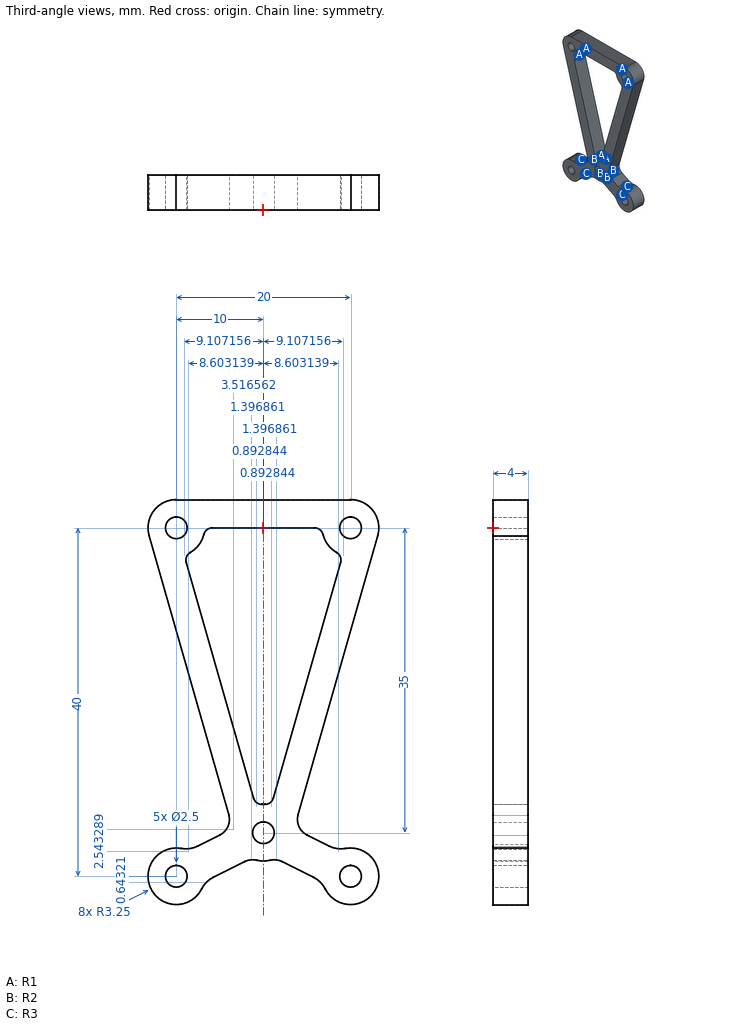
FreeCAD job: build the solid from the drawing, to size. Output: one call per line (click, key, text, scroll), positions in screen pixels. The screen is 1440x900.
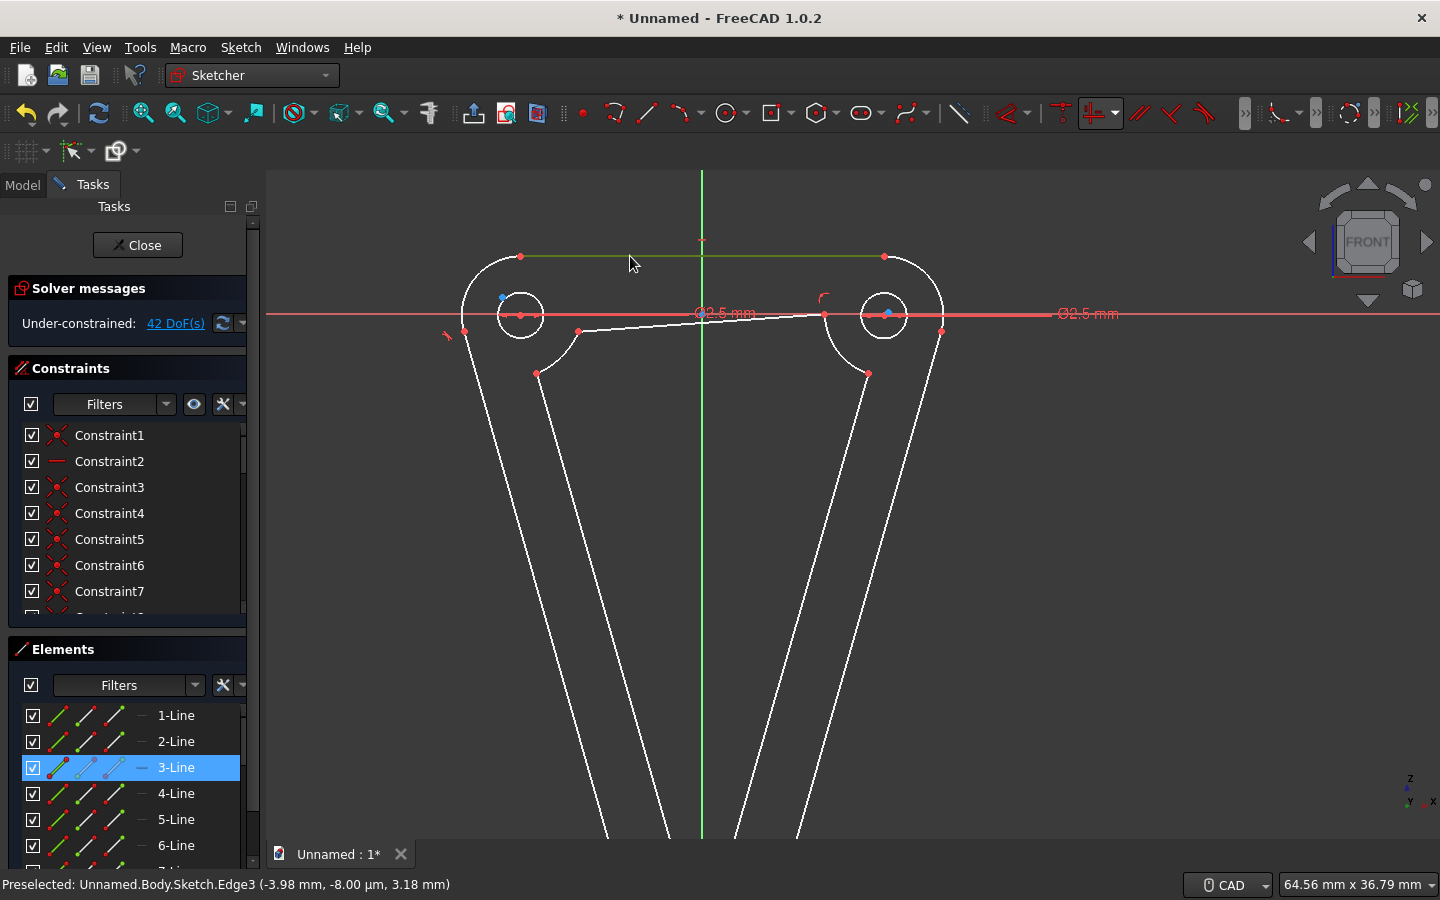
click(490, 265)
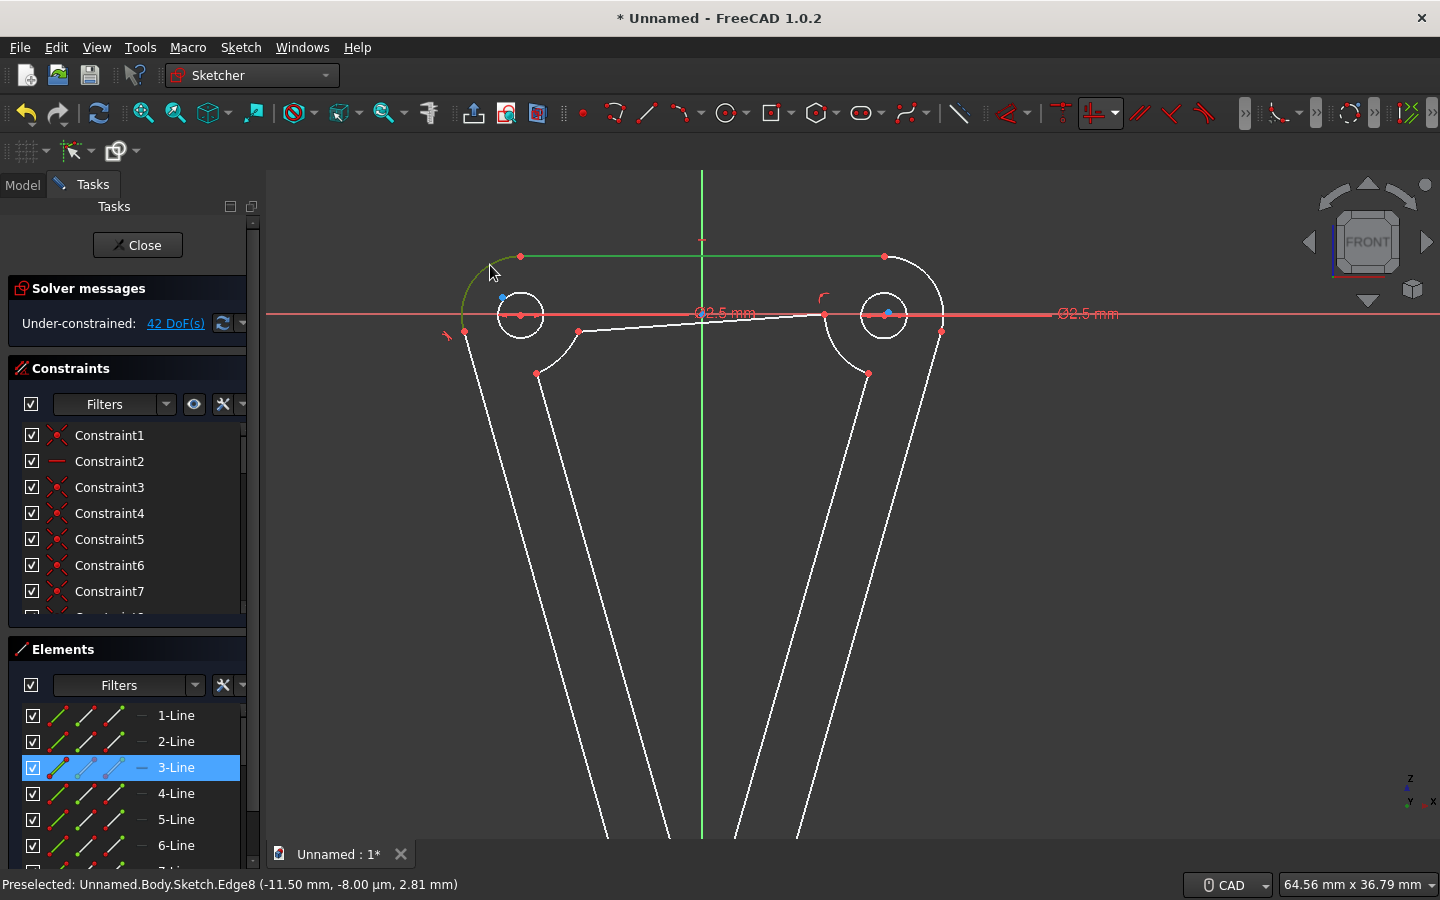
click(1204, 114)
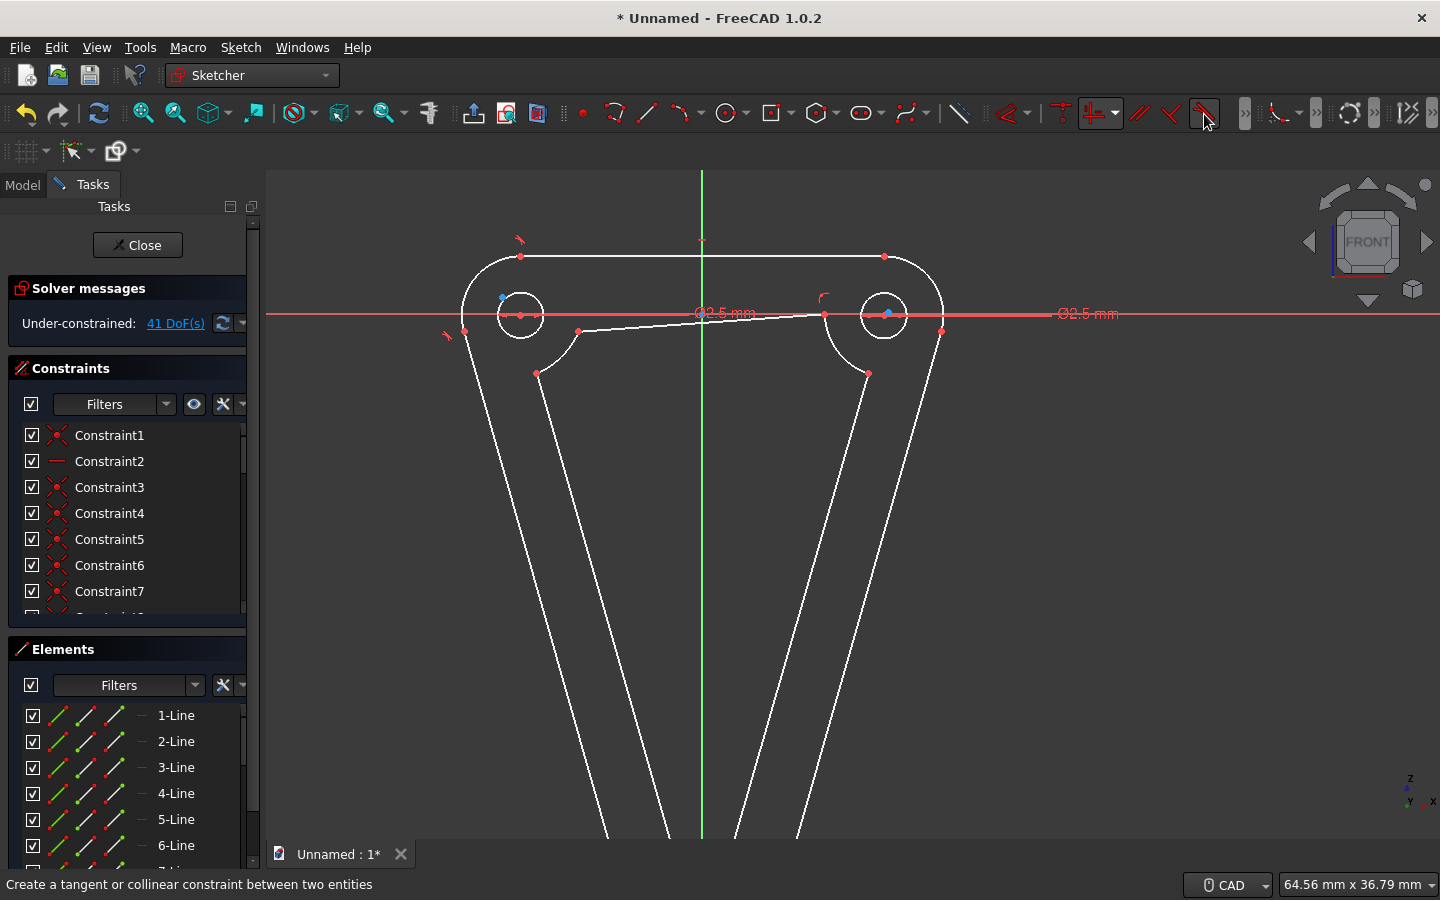
click(630, 256)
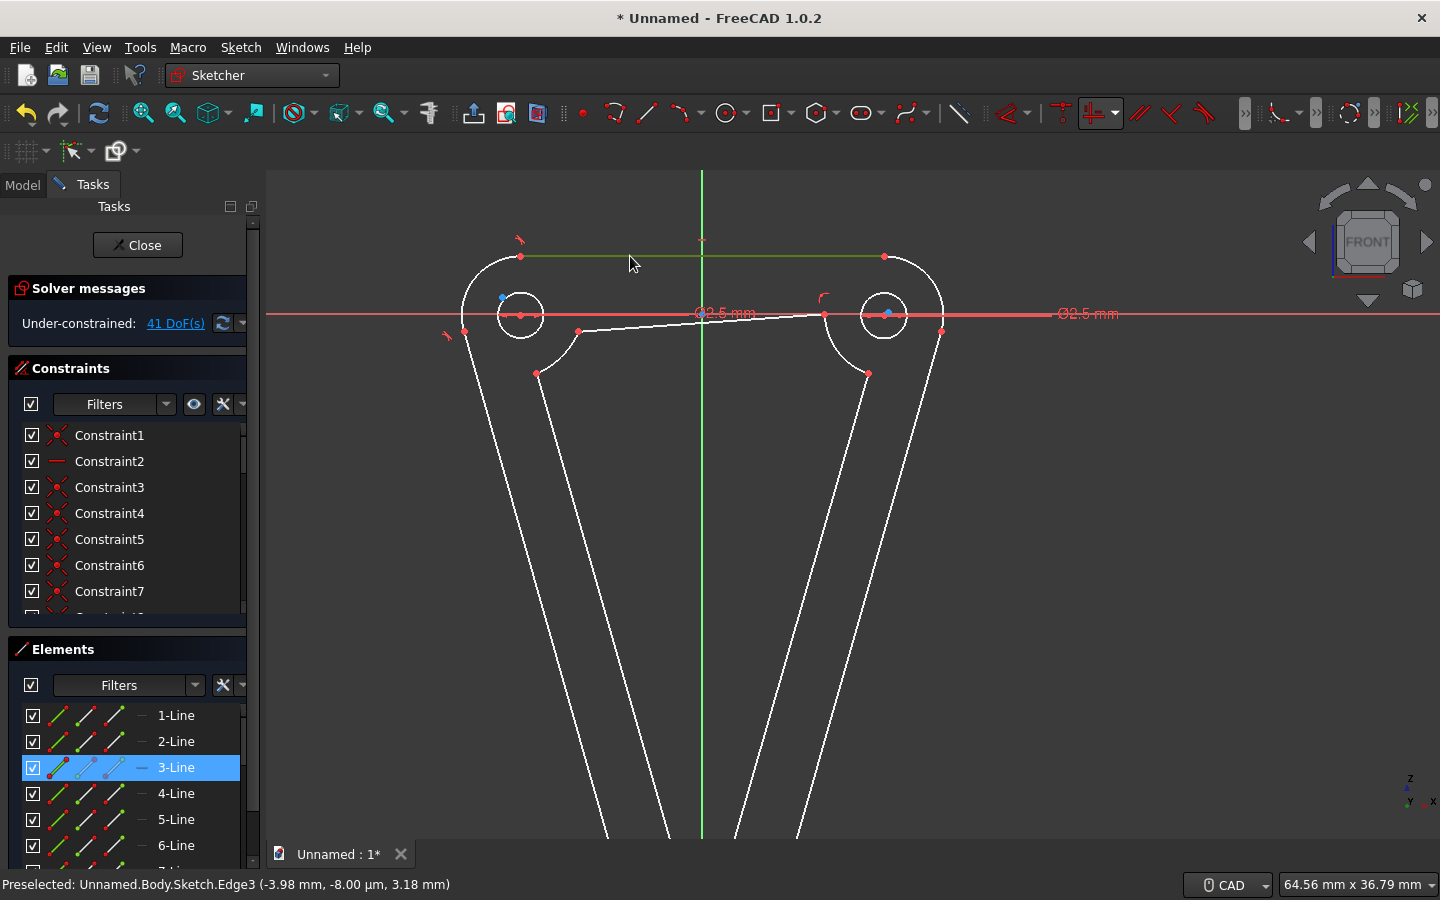
click(941, 299)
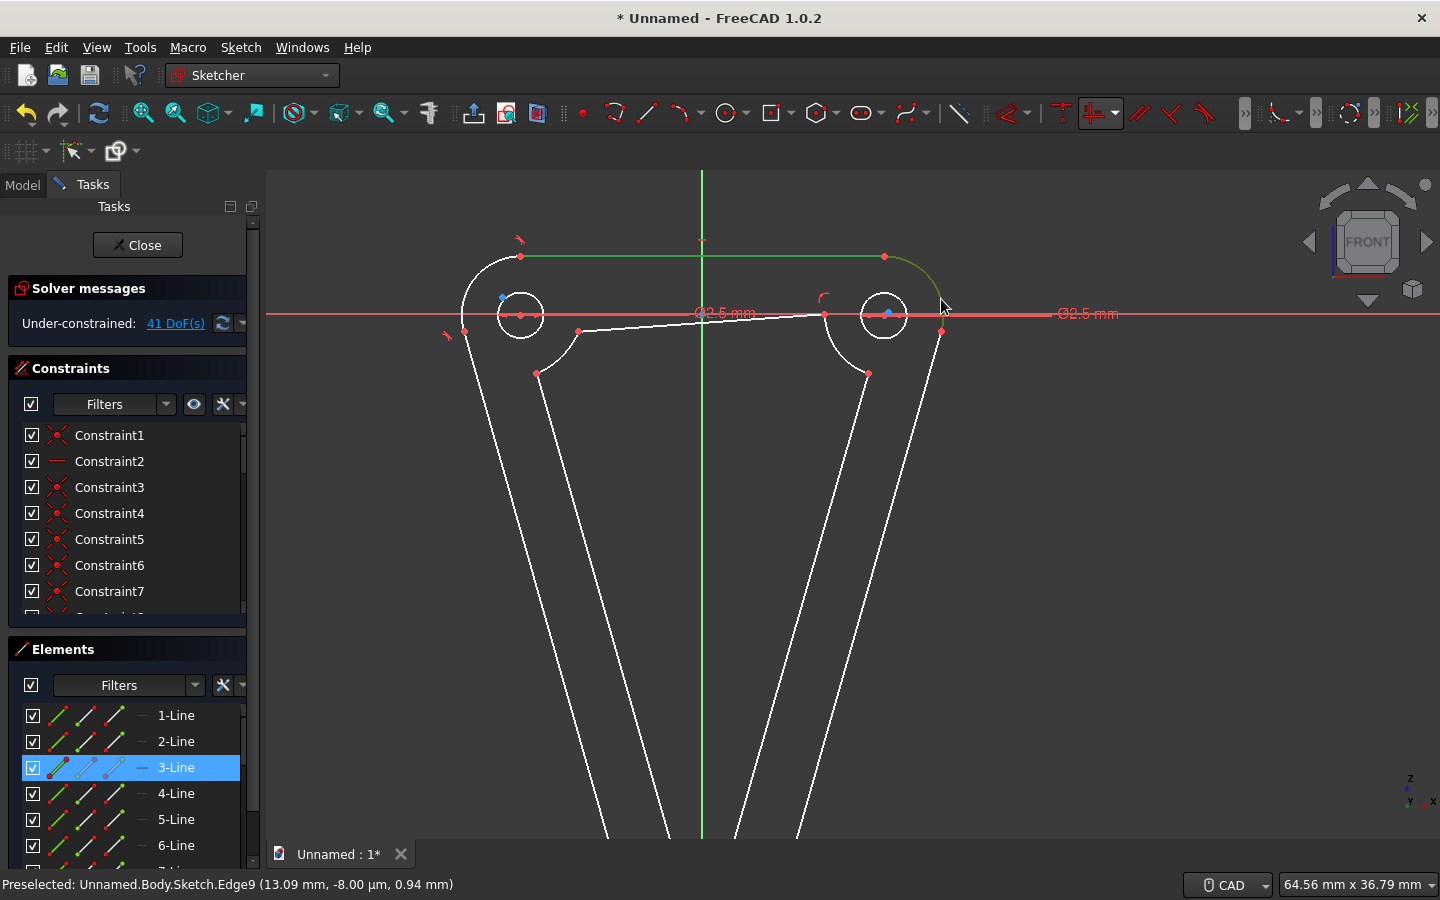
click(1204, 114)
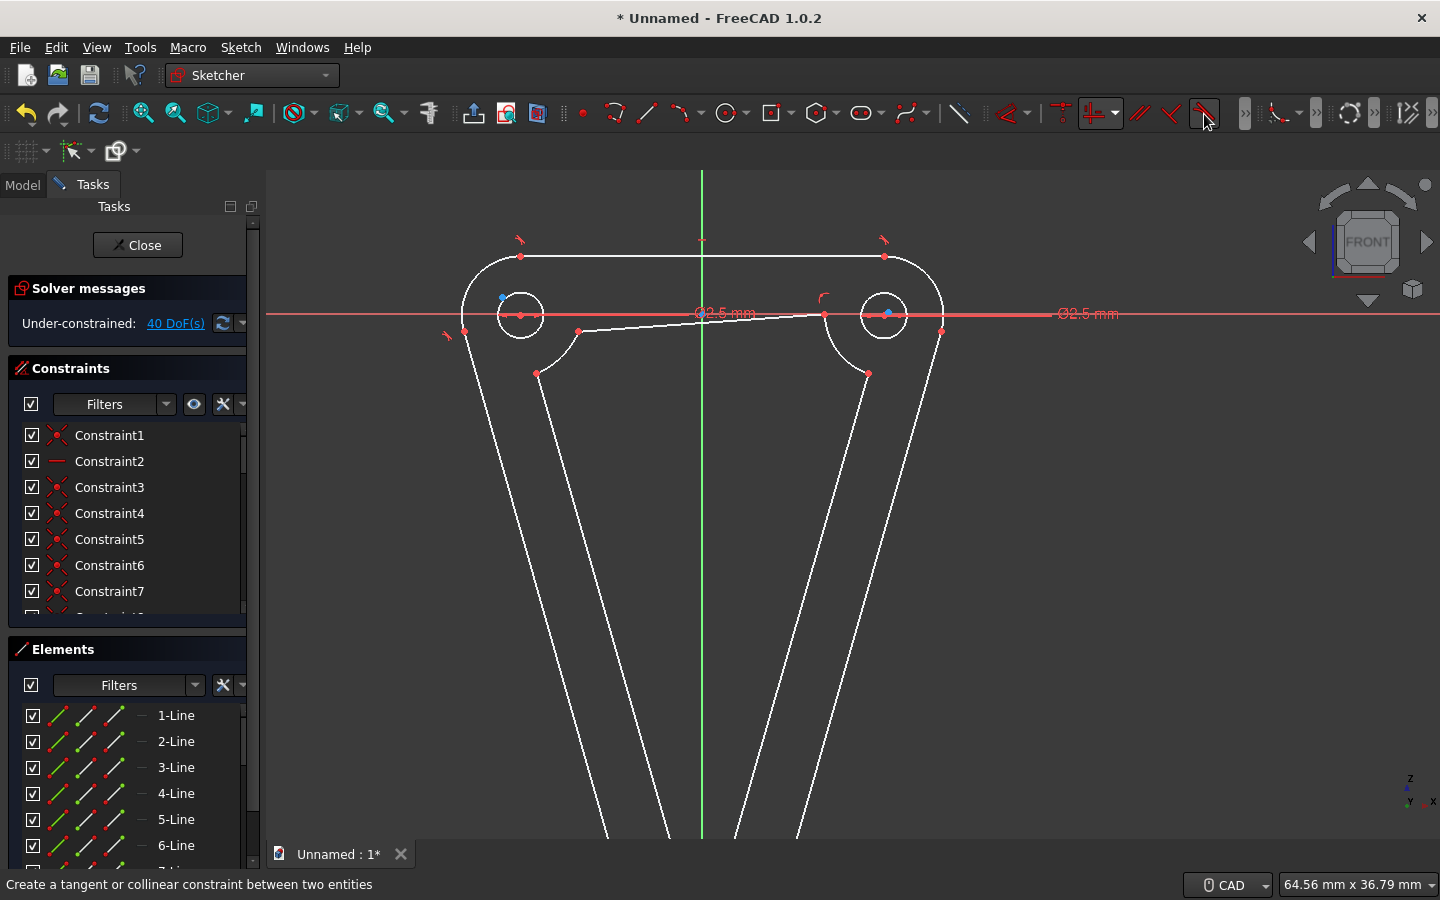
click(889, 515)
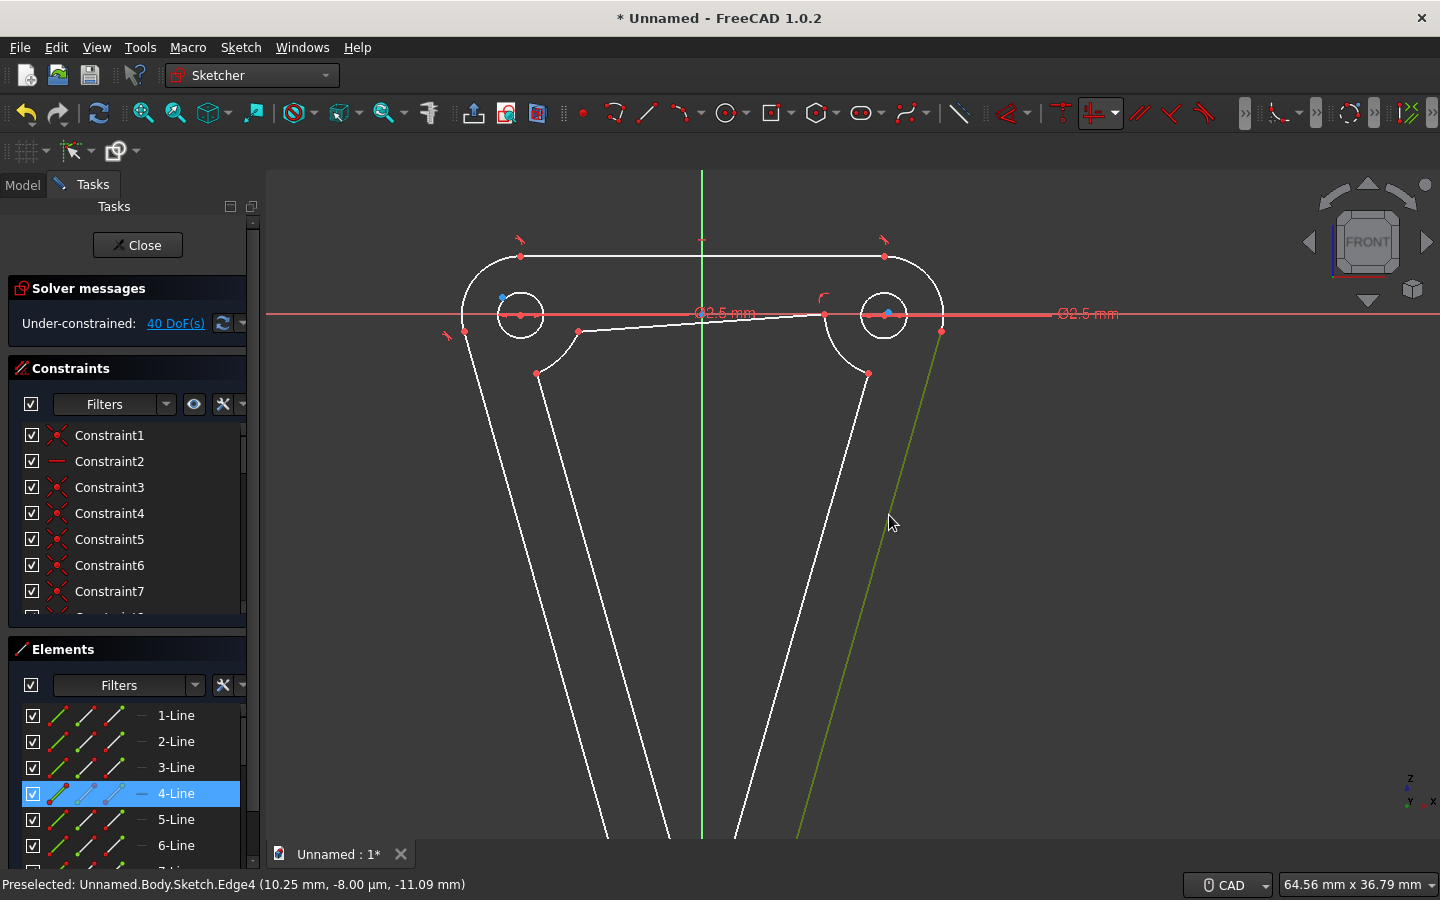
click(941, 299)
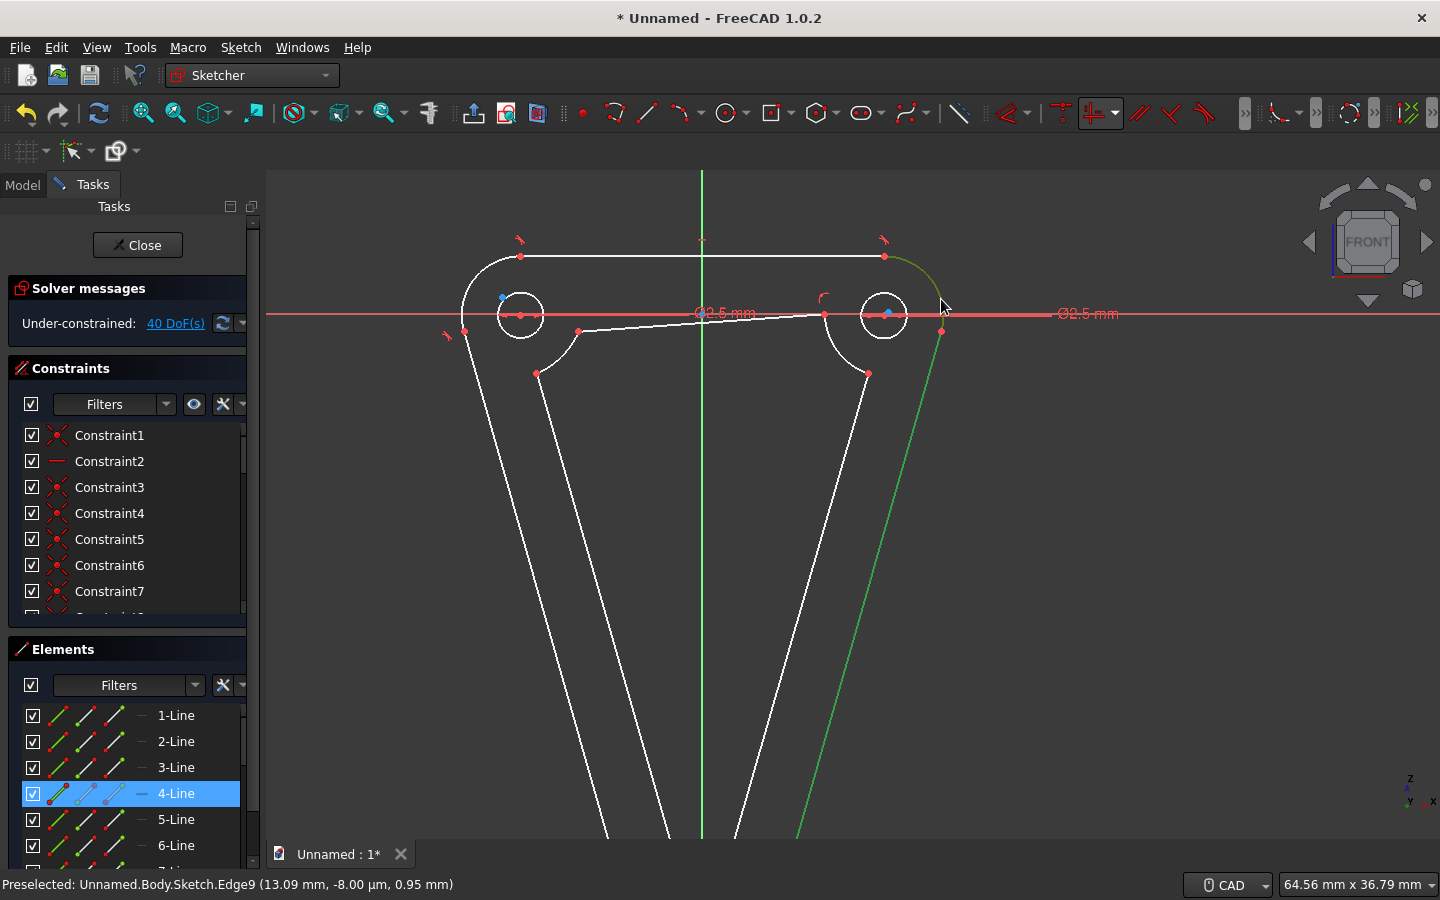
click(1204, 114)